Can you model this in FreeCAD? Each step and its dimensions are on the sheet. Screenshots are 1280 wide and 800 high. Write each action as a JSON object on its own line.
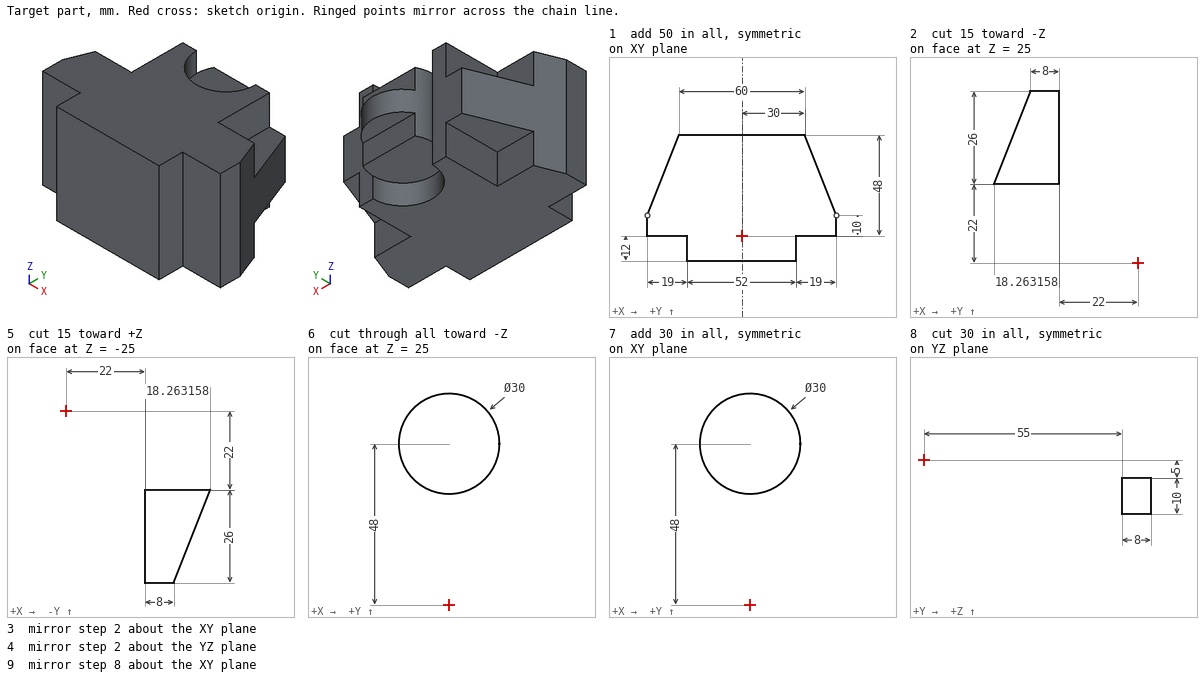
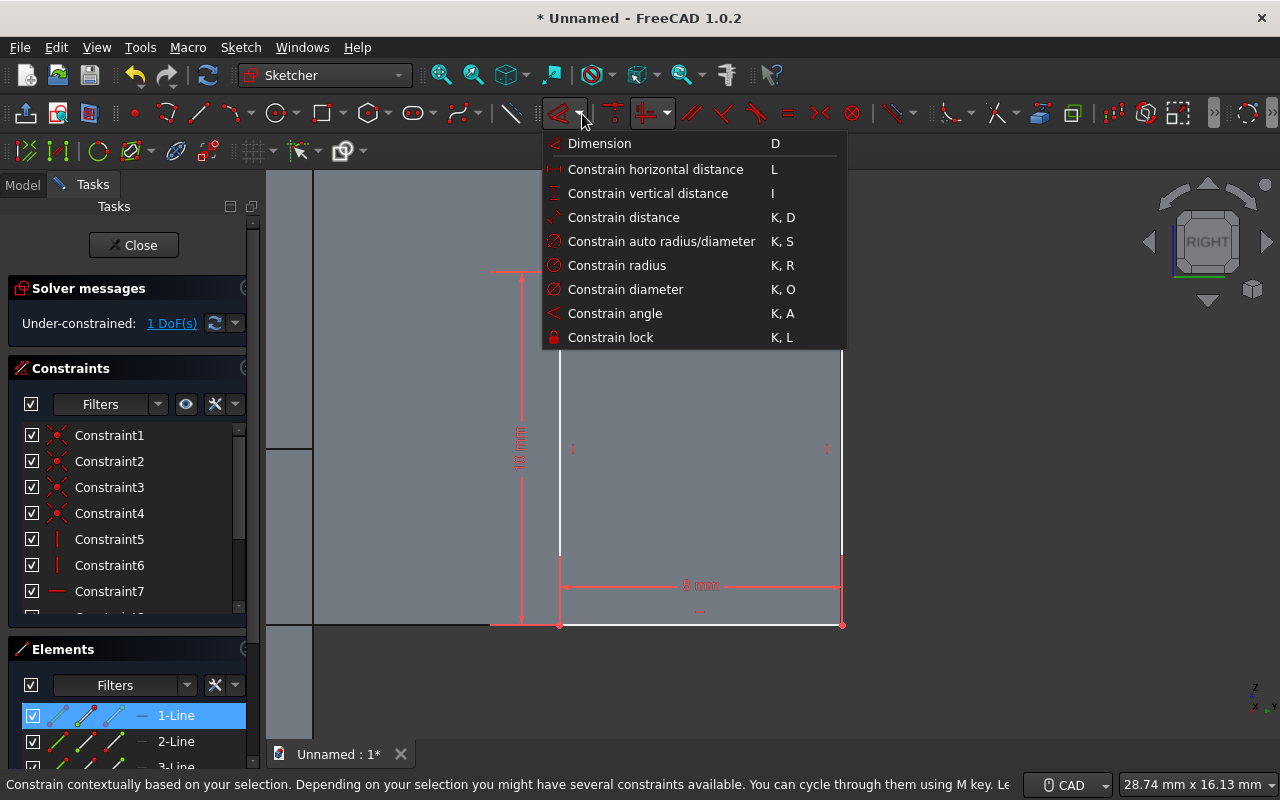
{"action": "left_click", "coordinate": [695, 169]}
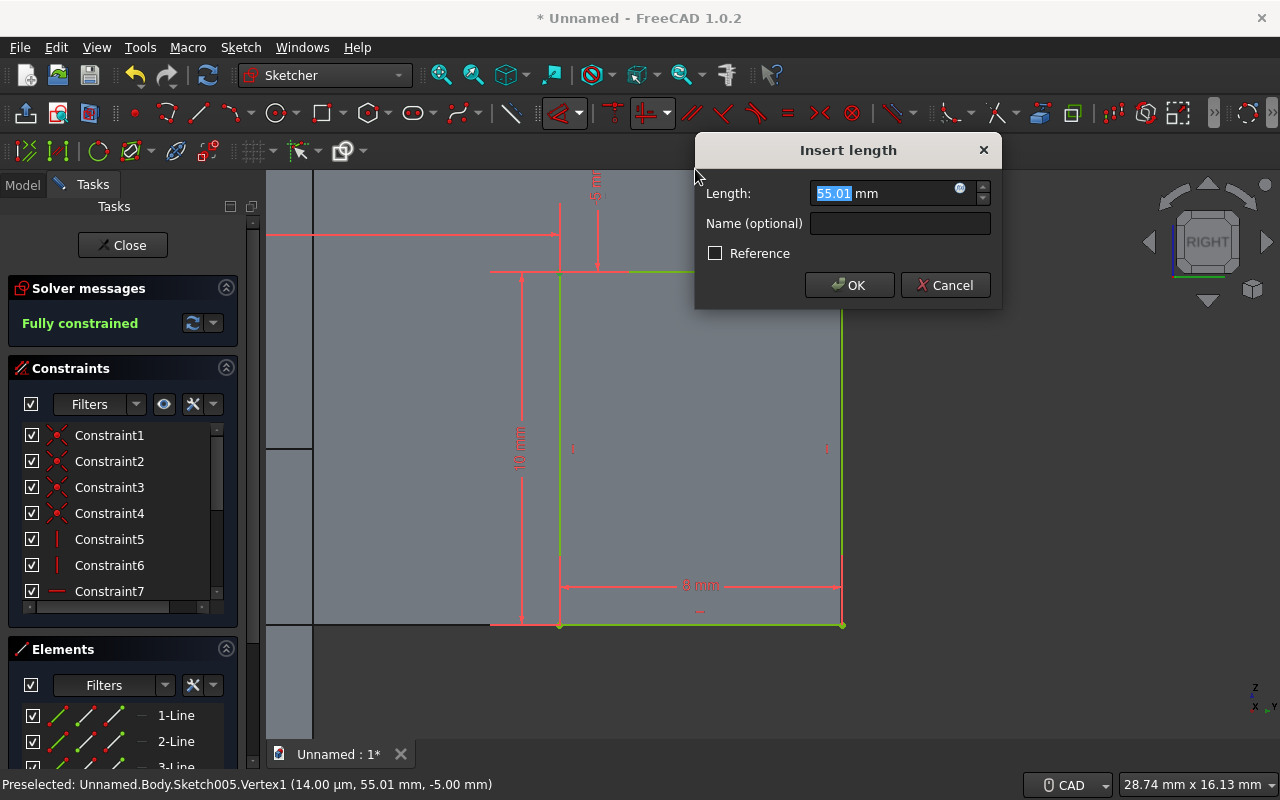
{"action": "type", "text": "55"}
{"action": "key", "text": "Return"}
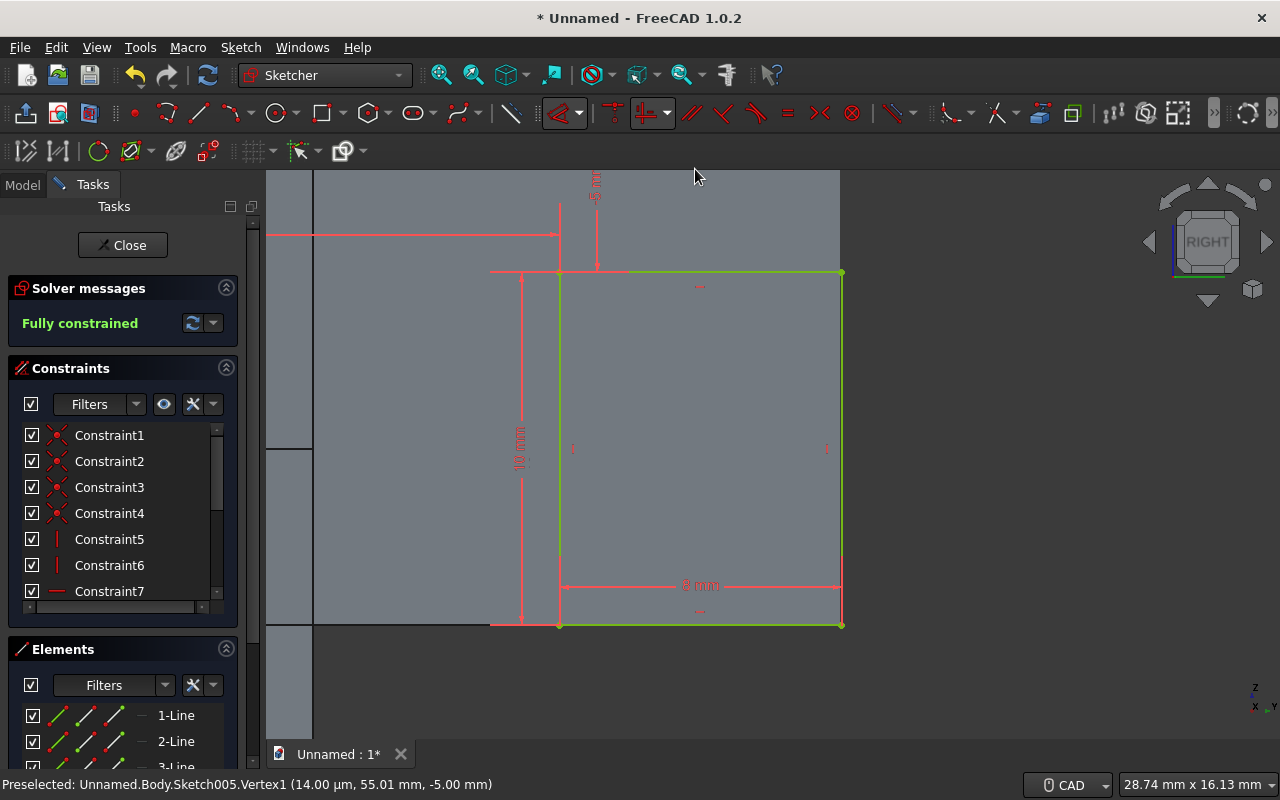
{"action": "left_click", "coordinate": [123, 245]}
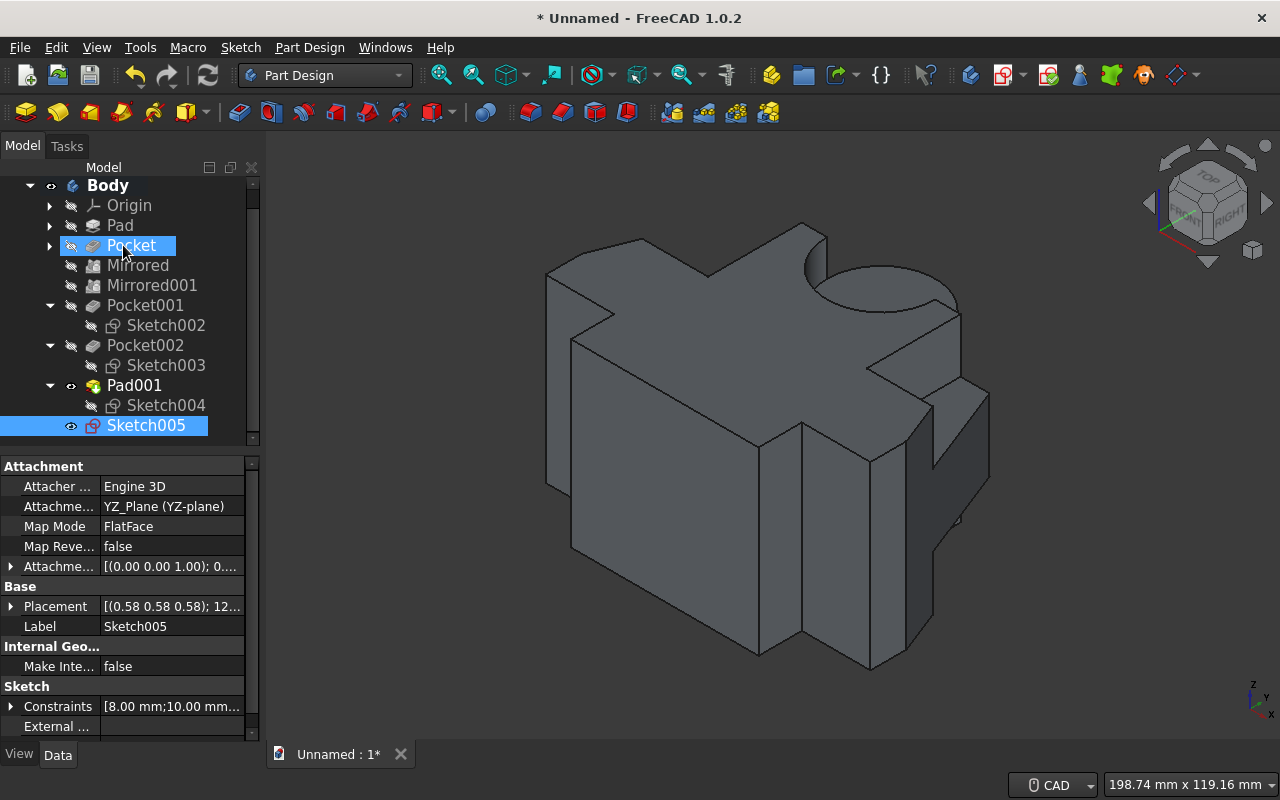
{"action": "left_click", "coordinate": [240, 112]}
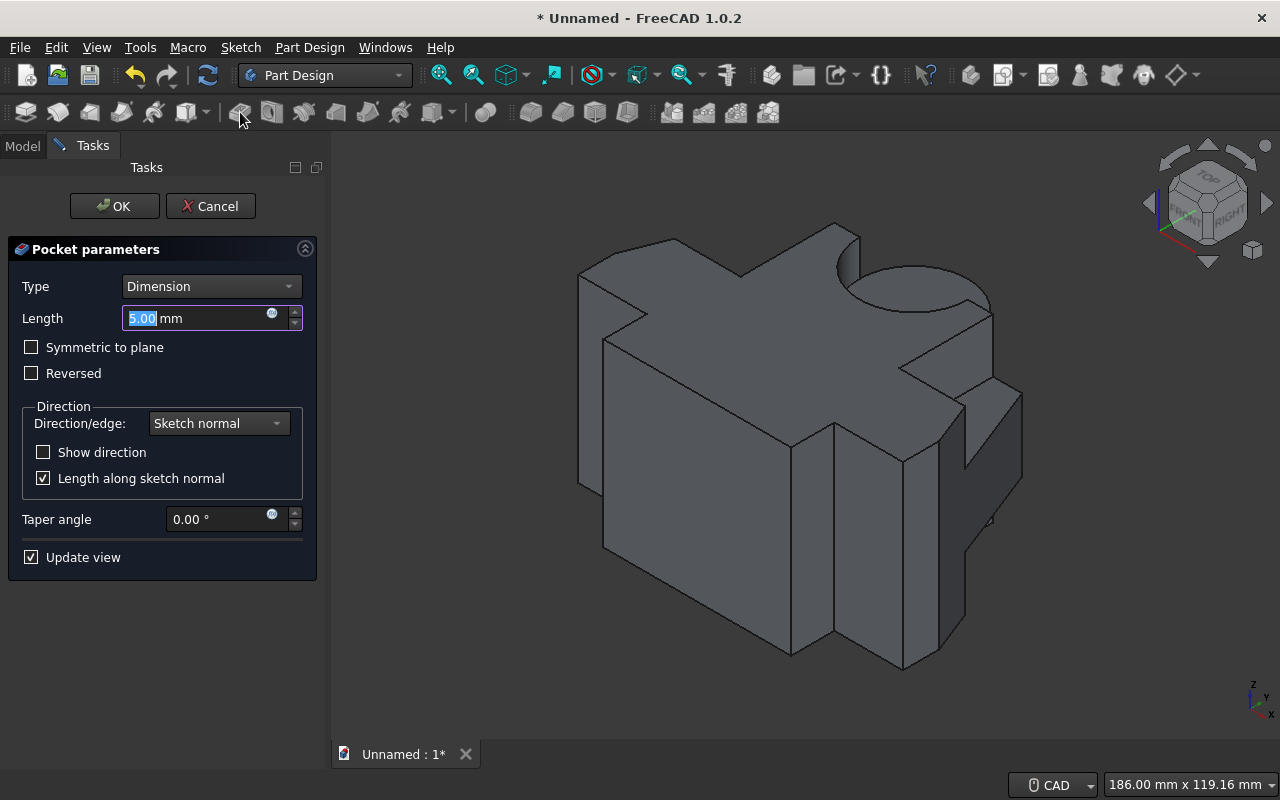
{"action": "type", "text": "30"}
{"action": "key", "text": "Tab"}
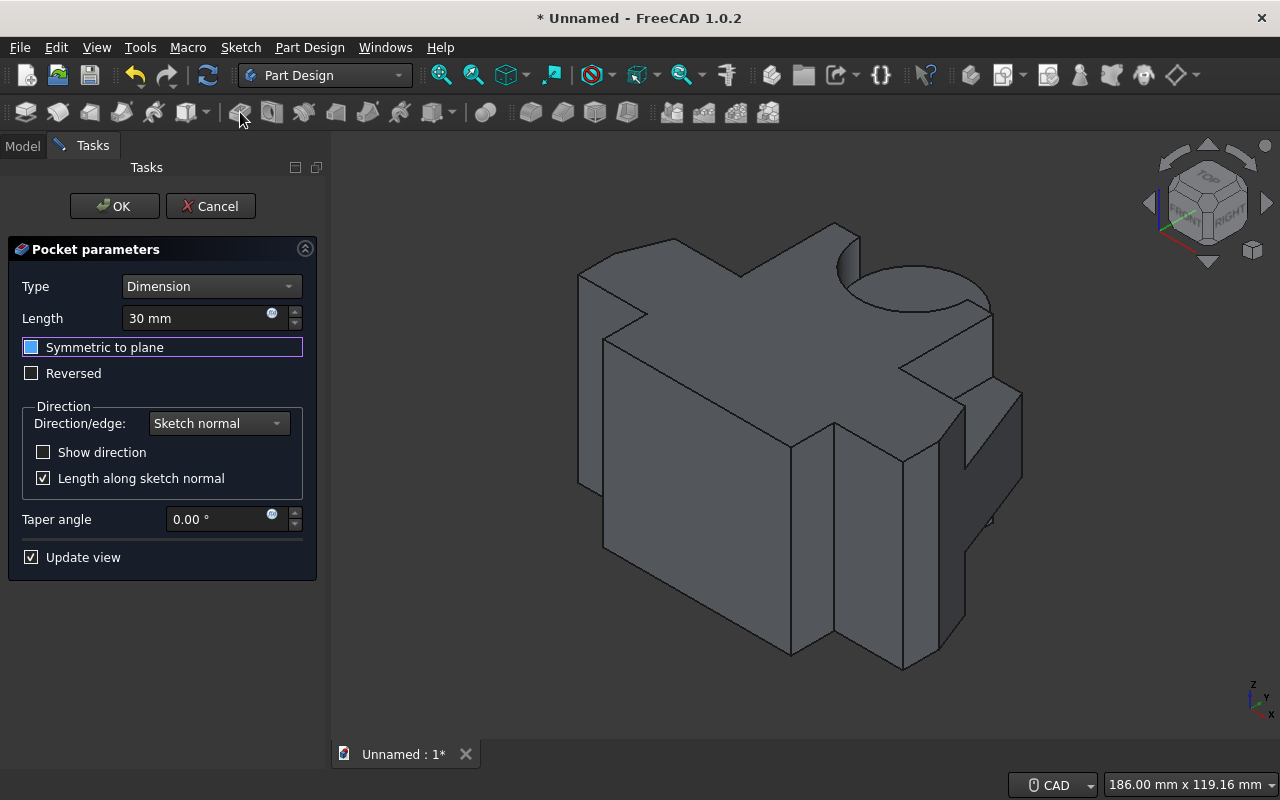
{"action": "left_click", "coordinate": [30, 347]}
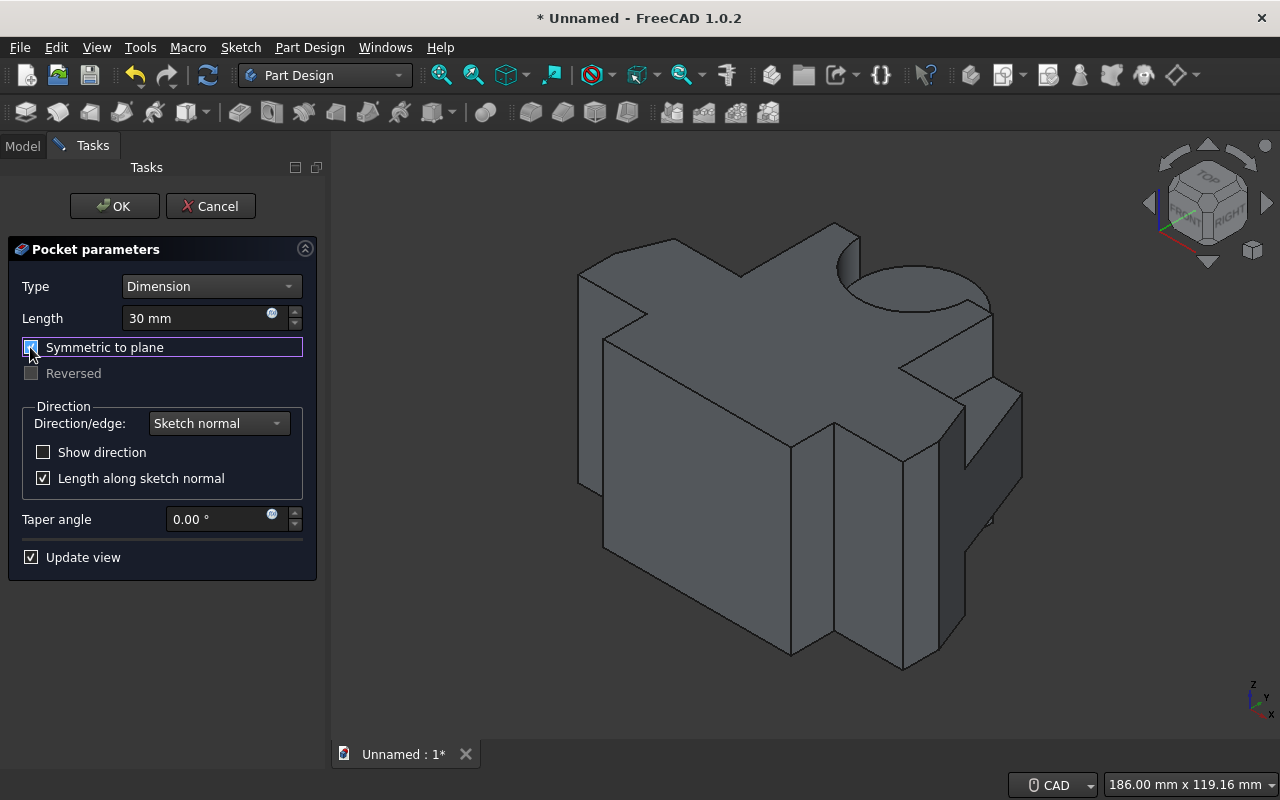
{"action": "left_click", "coordinate": [115, 206]}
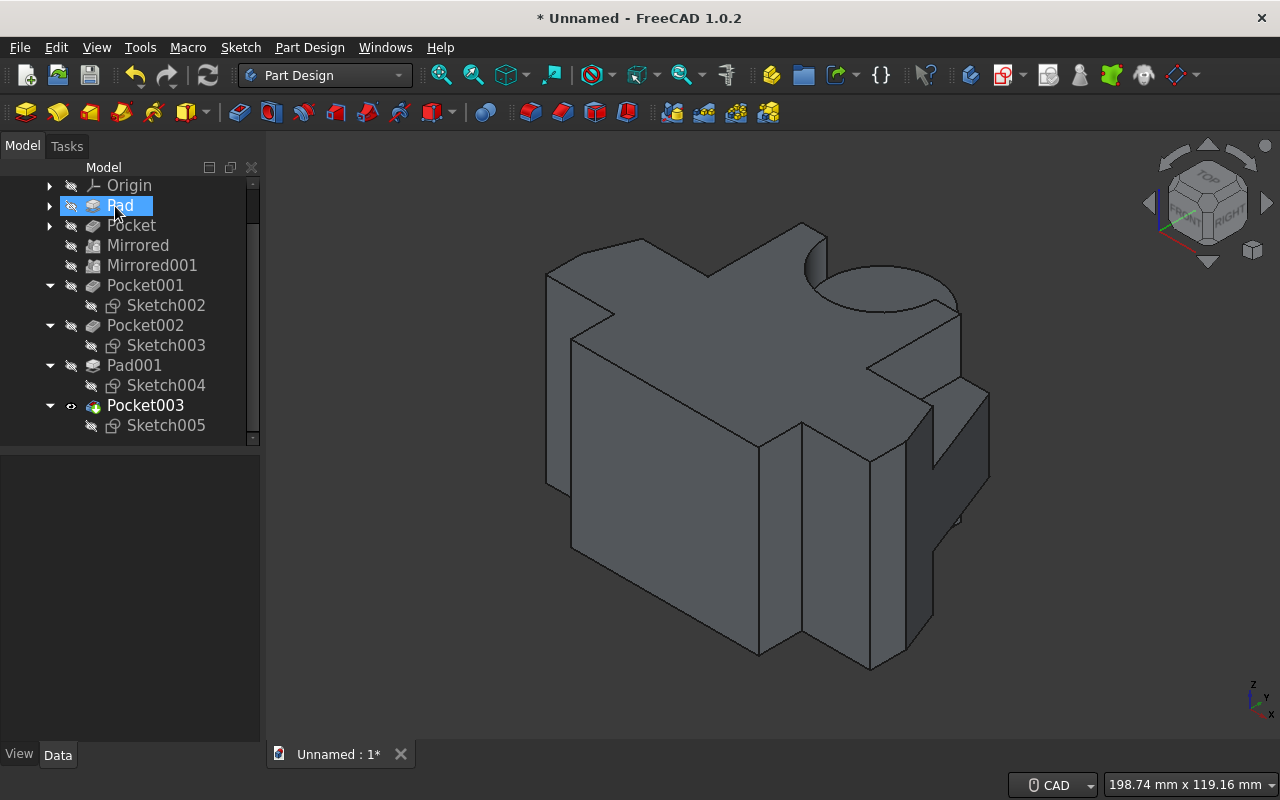
{"action": "left_click", "coordinate": [116, 406]}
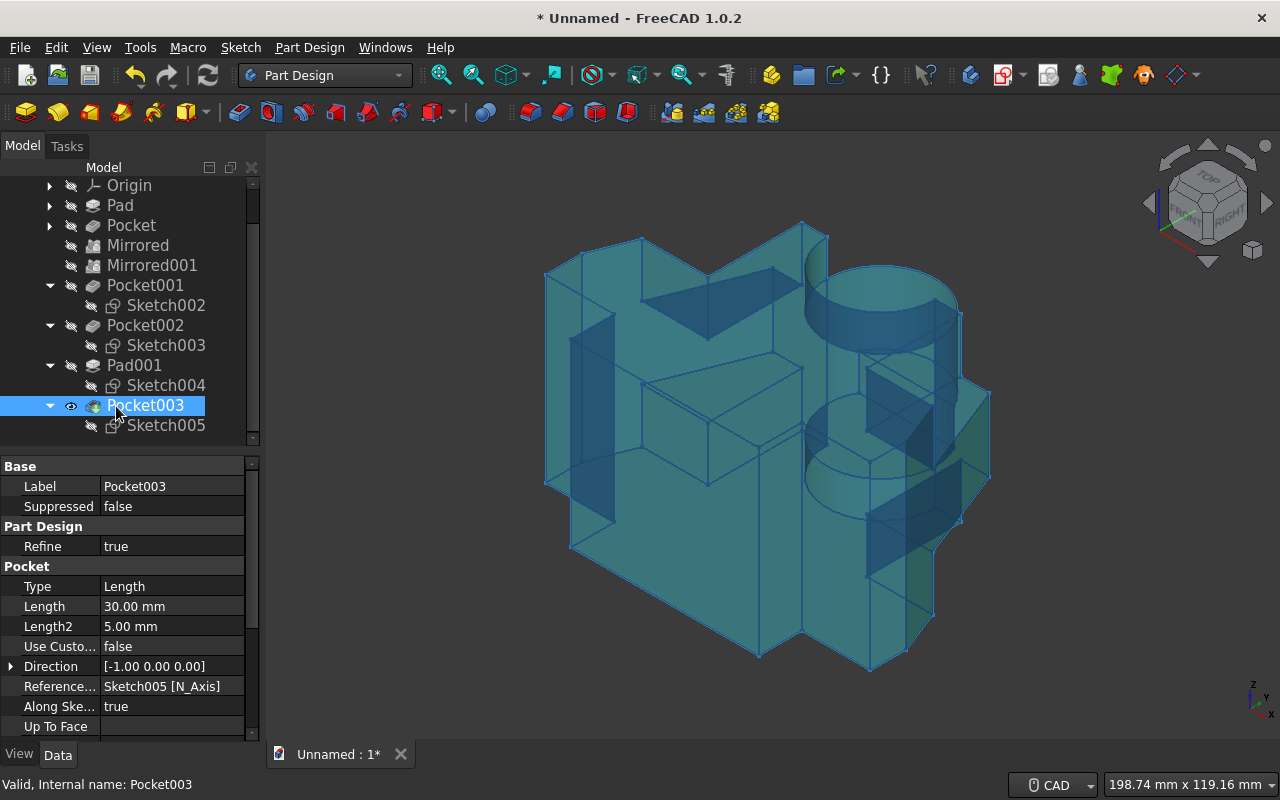
{"action": "left_click", "coordinate": [672, 112]}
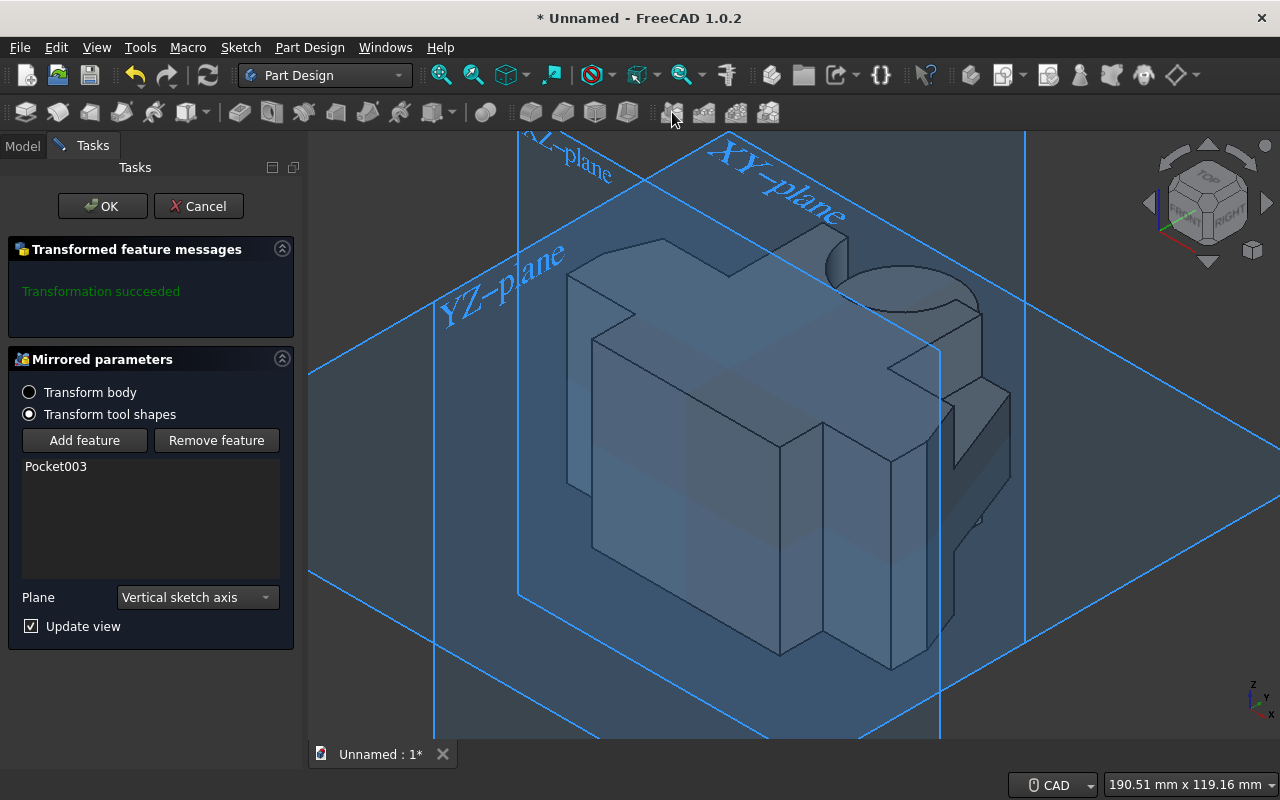
{"action": "left_click", "coordinate": [198, 598]}